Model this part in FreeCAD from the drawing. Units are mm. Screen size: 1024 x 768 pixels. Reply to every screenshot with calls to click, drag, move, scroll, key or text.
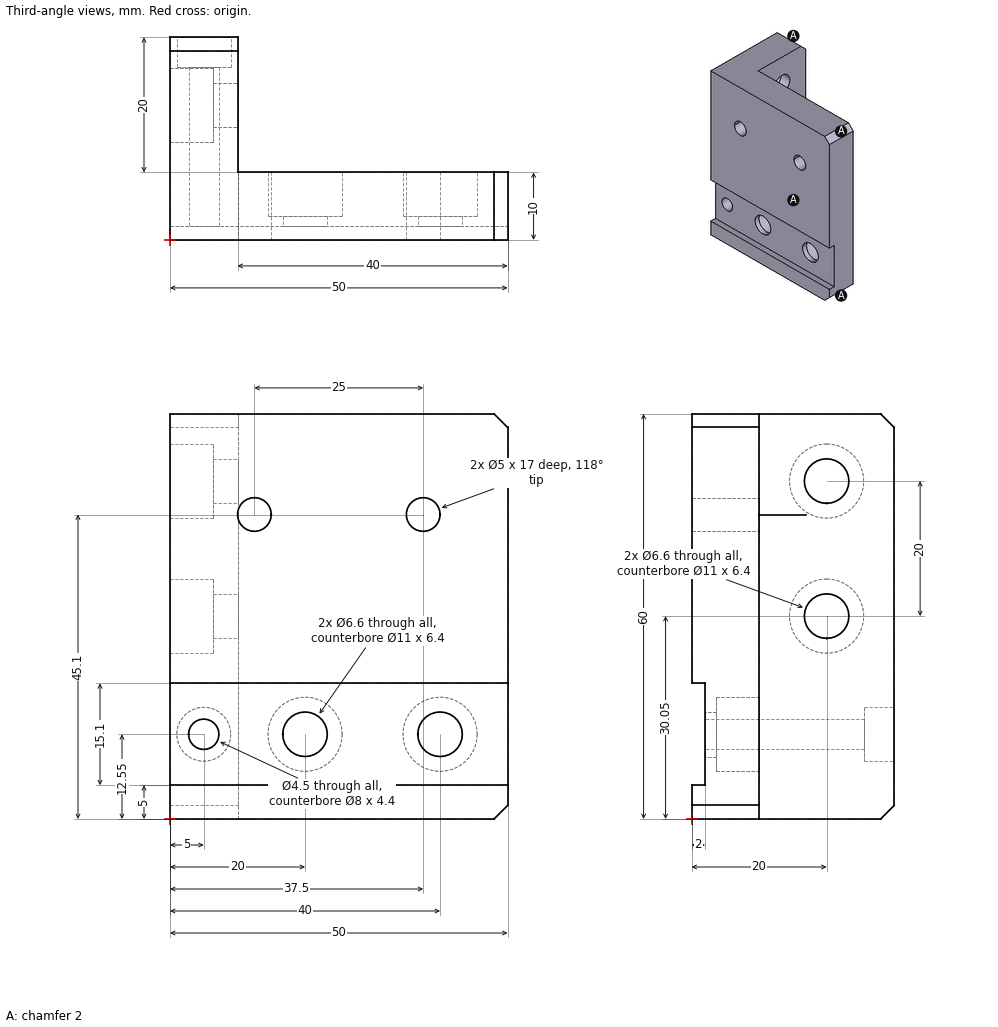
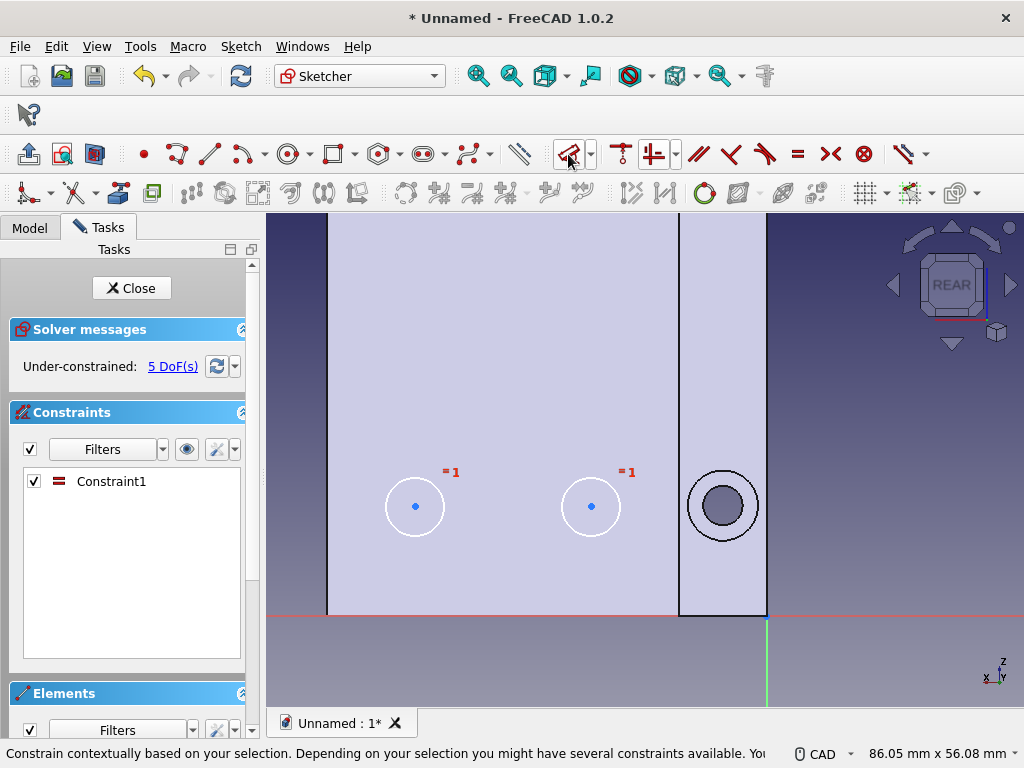
click(611, 486)
click(633, 463)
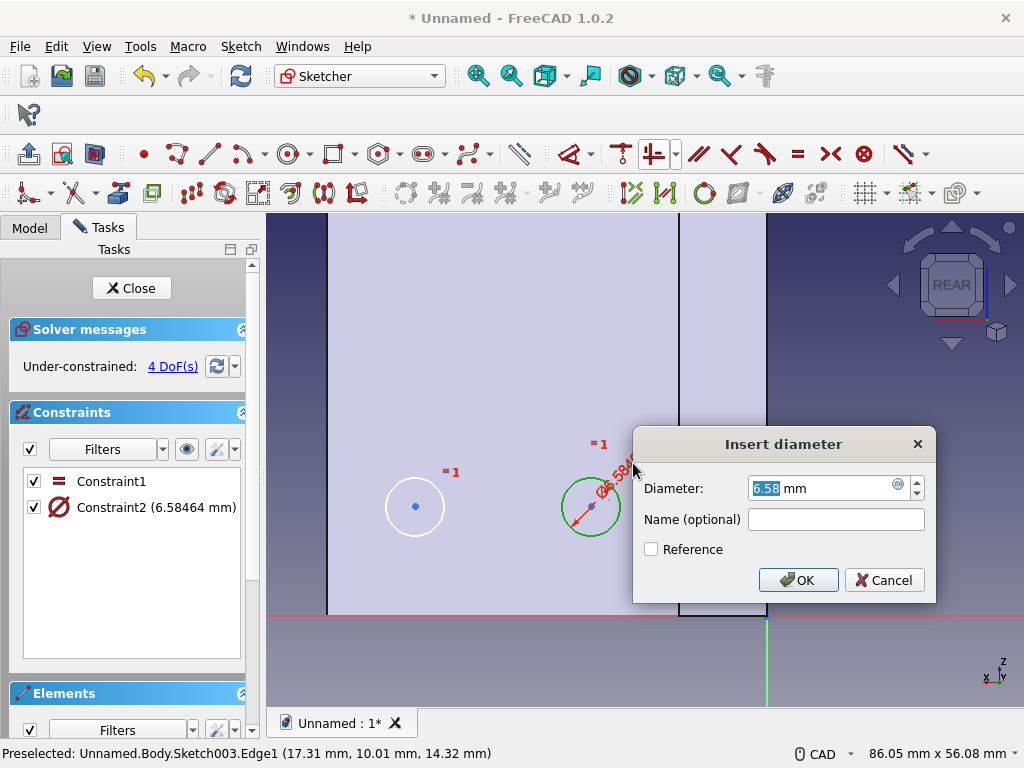
text(6.6)
key(Return)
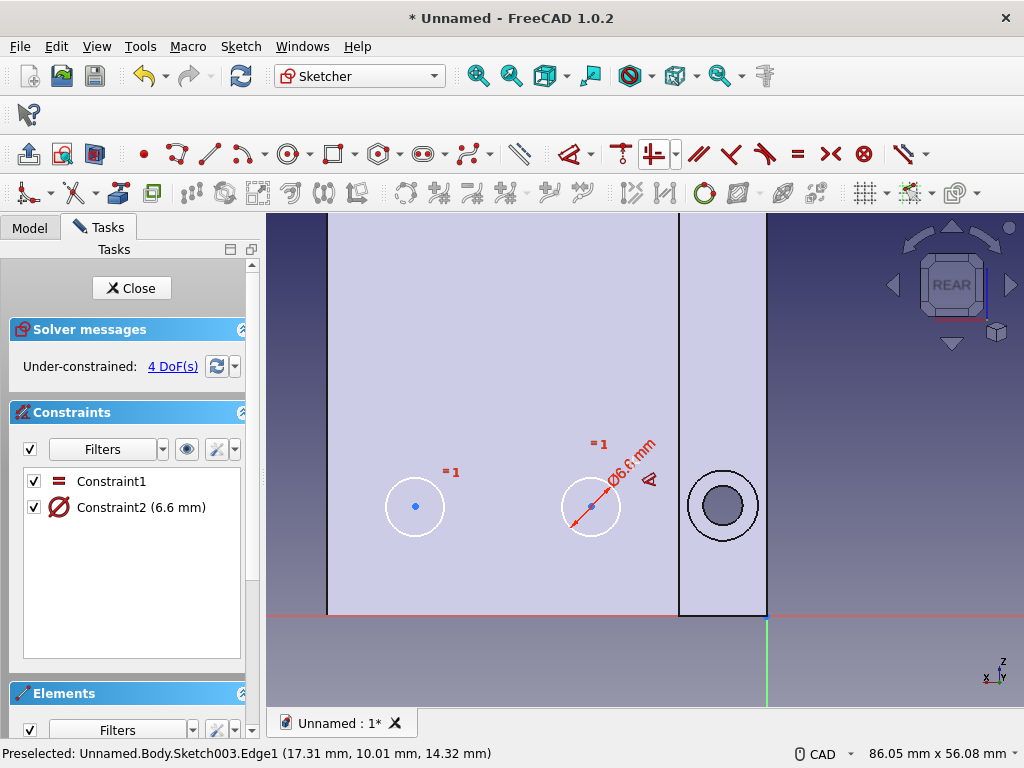
click(591, 507)
click(679, 650)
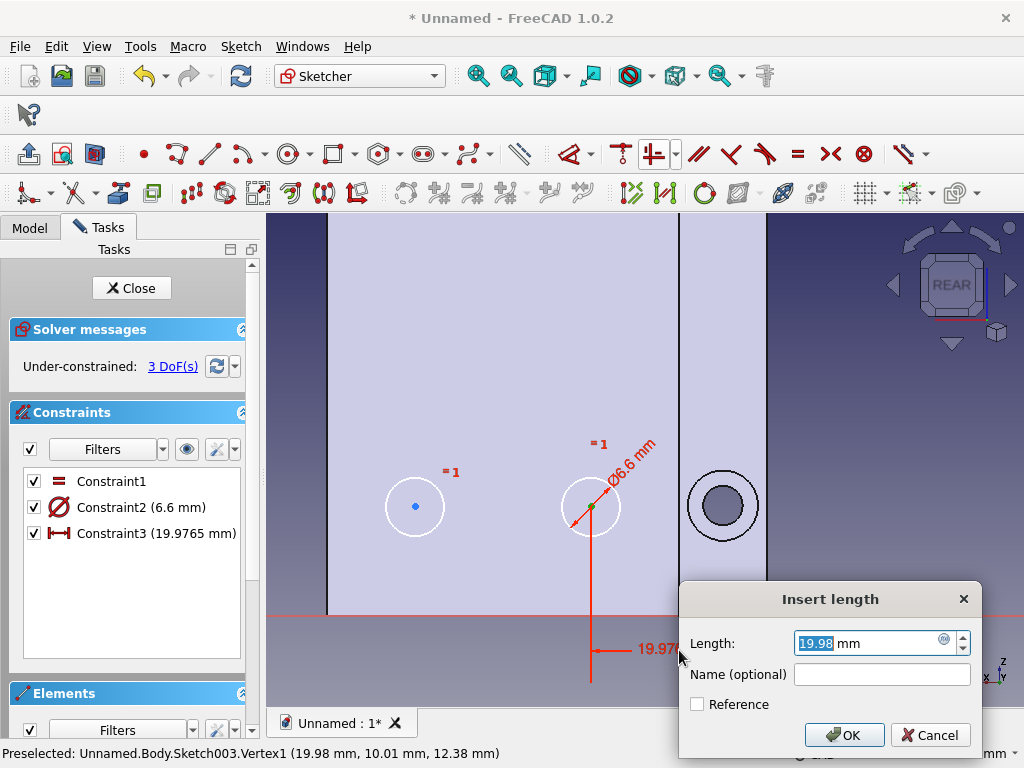
text(20)
key(Return)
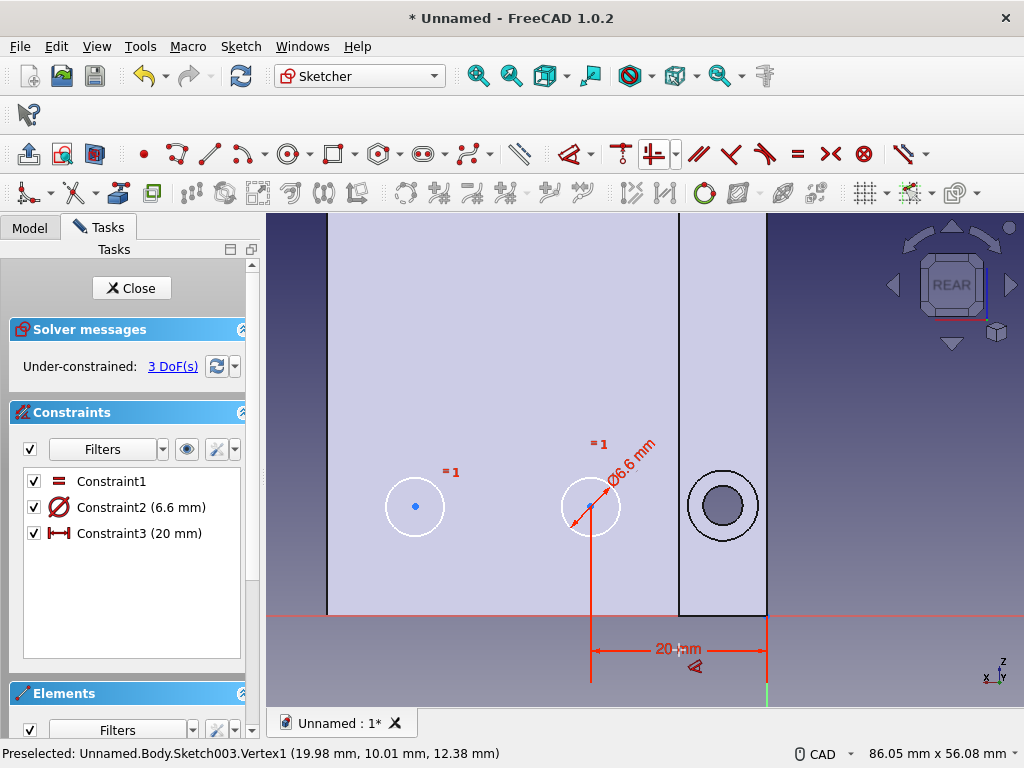
click(415, 507)
click(591, 650)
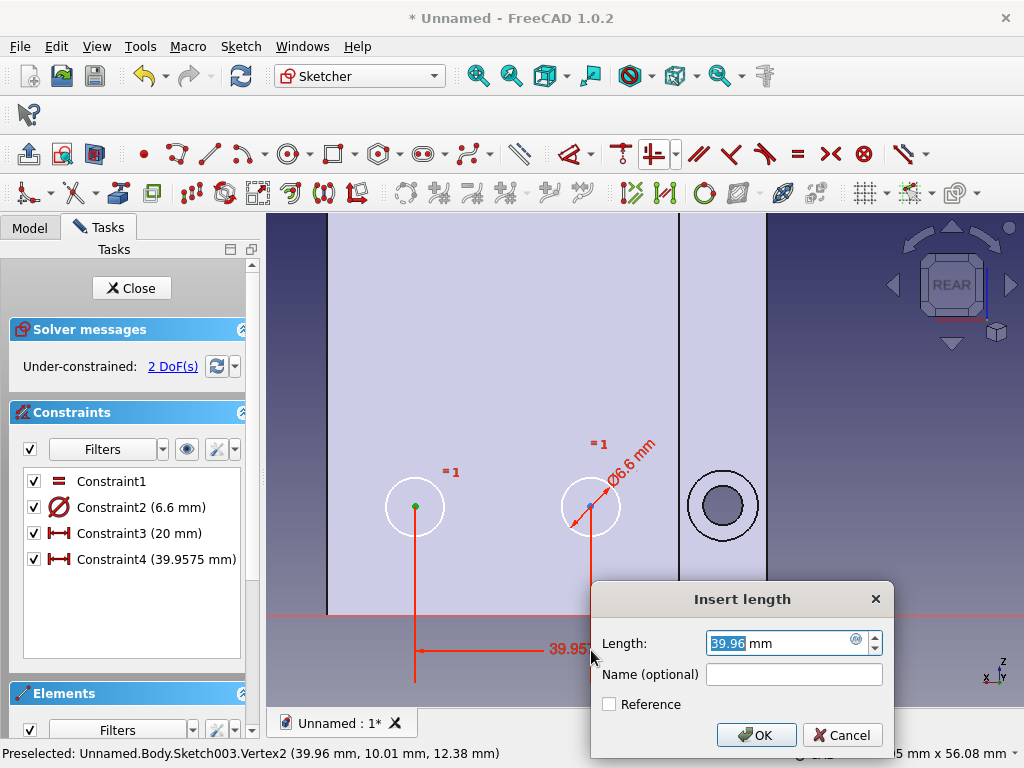
text(40)
key(Return)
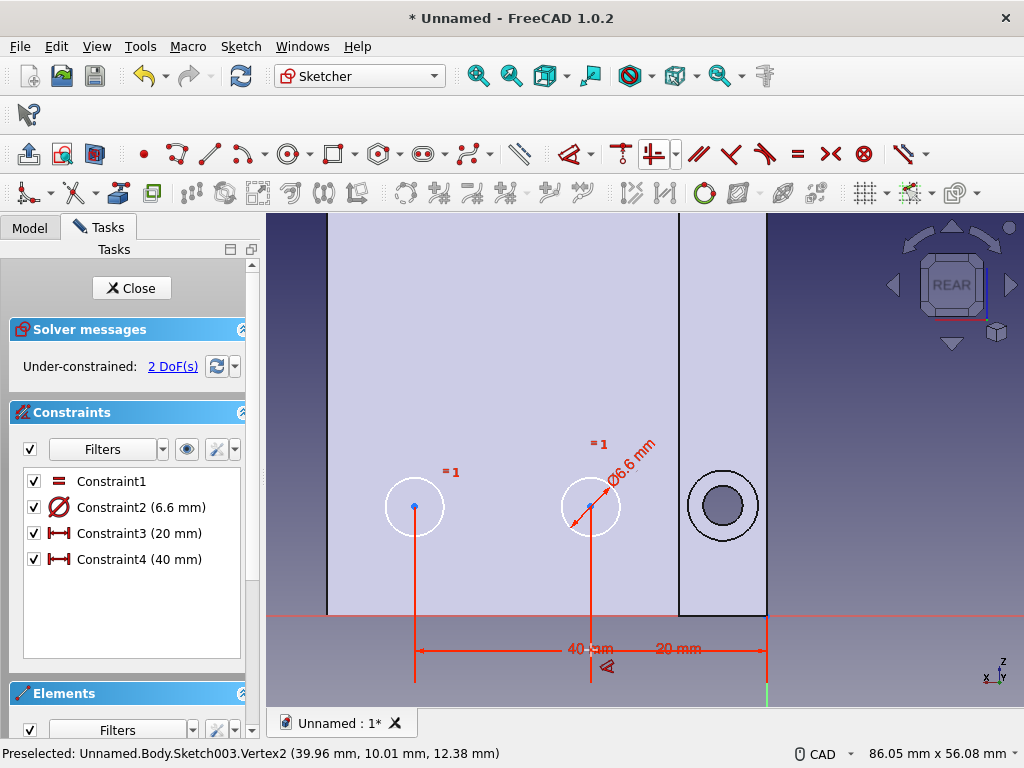
click(591, 507)
click(801, 562)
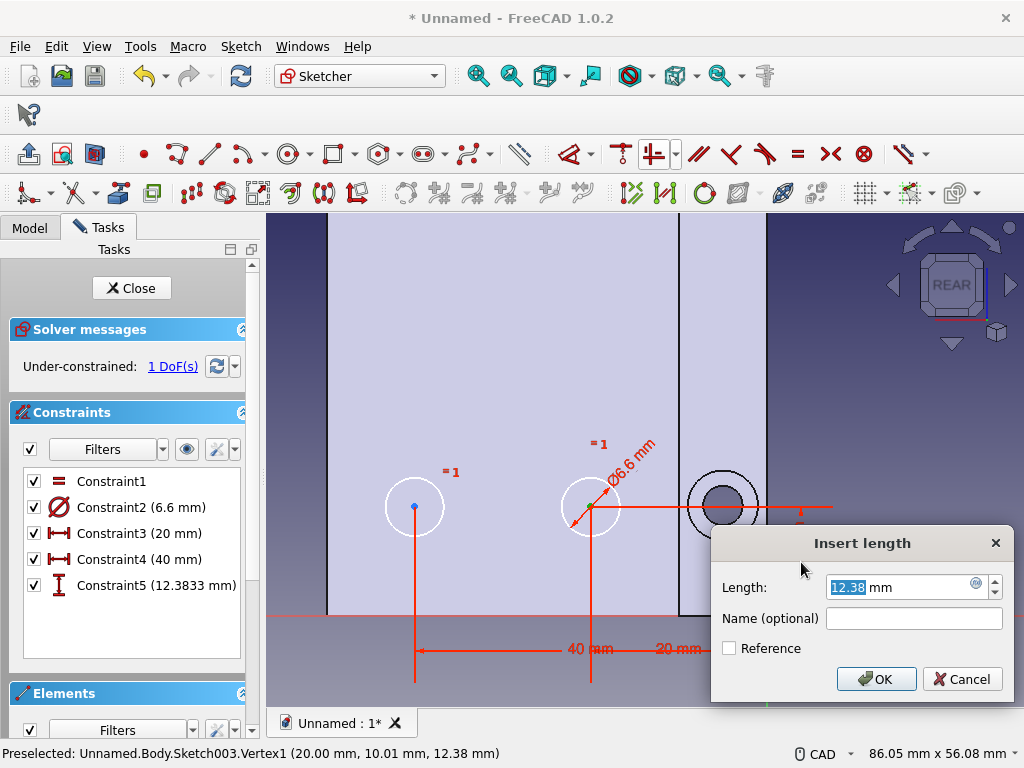
text(12.55)
key(Return)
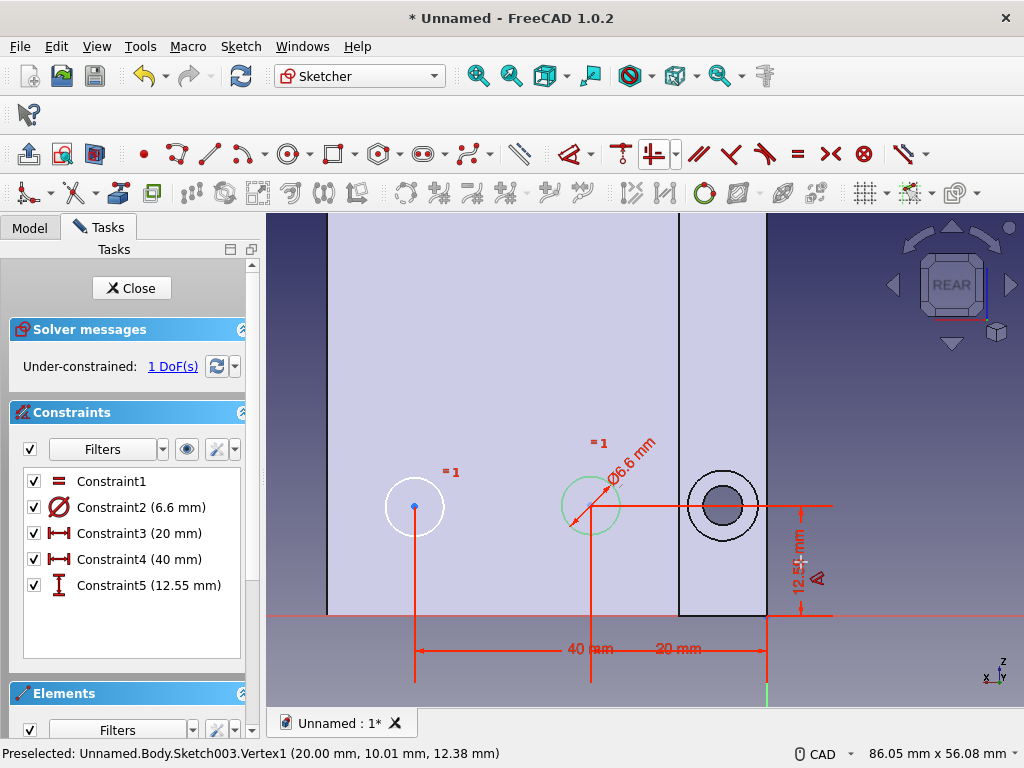
click(415, 507)
click(801, 536)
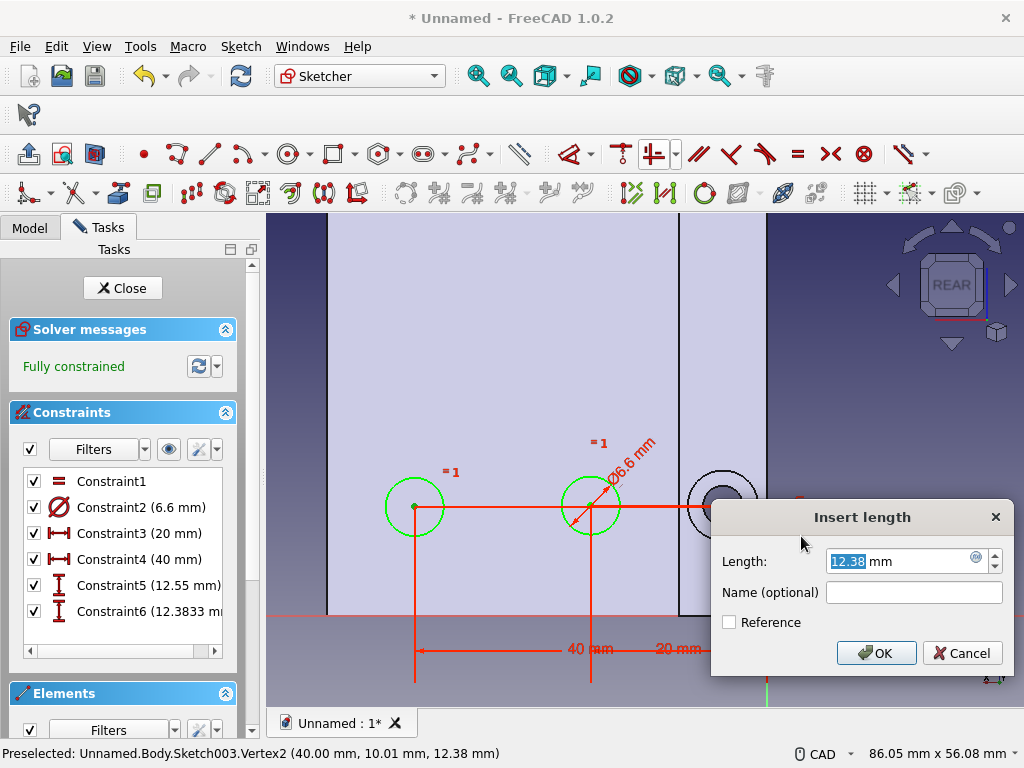
text(12.55)
key(Return)
key(Escape)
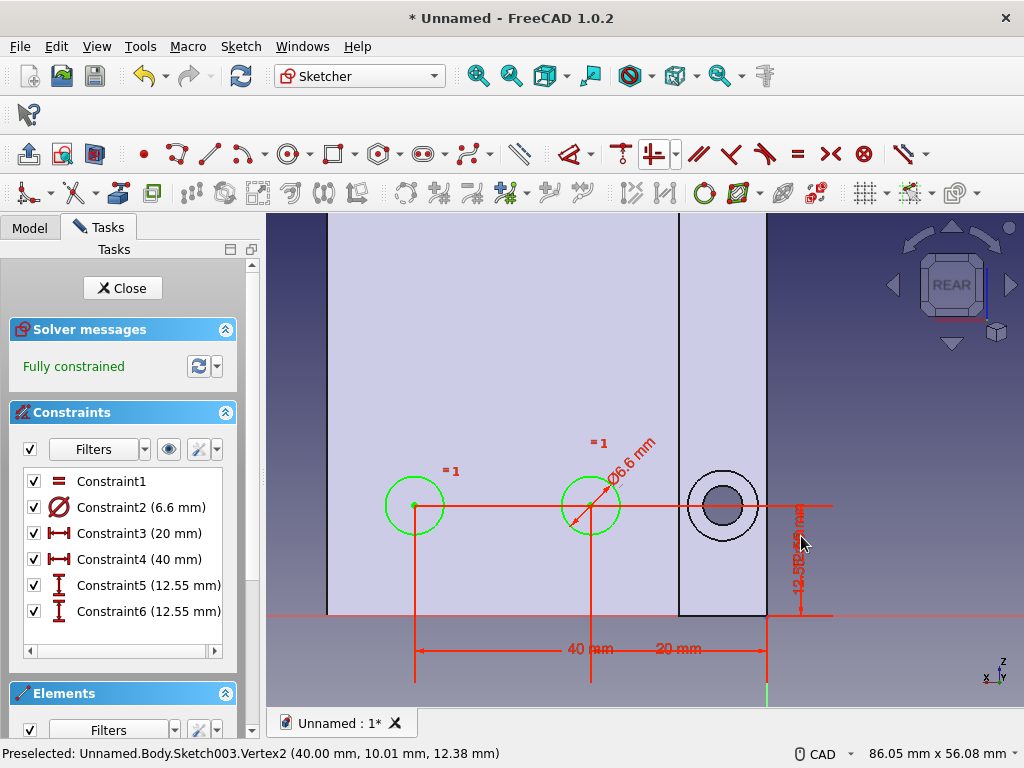
click(123, 288)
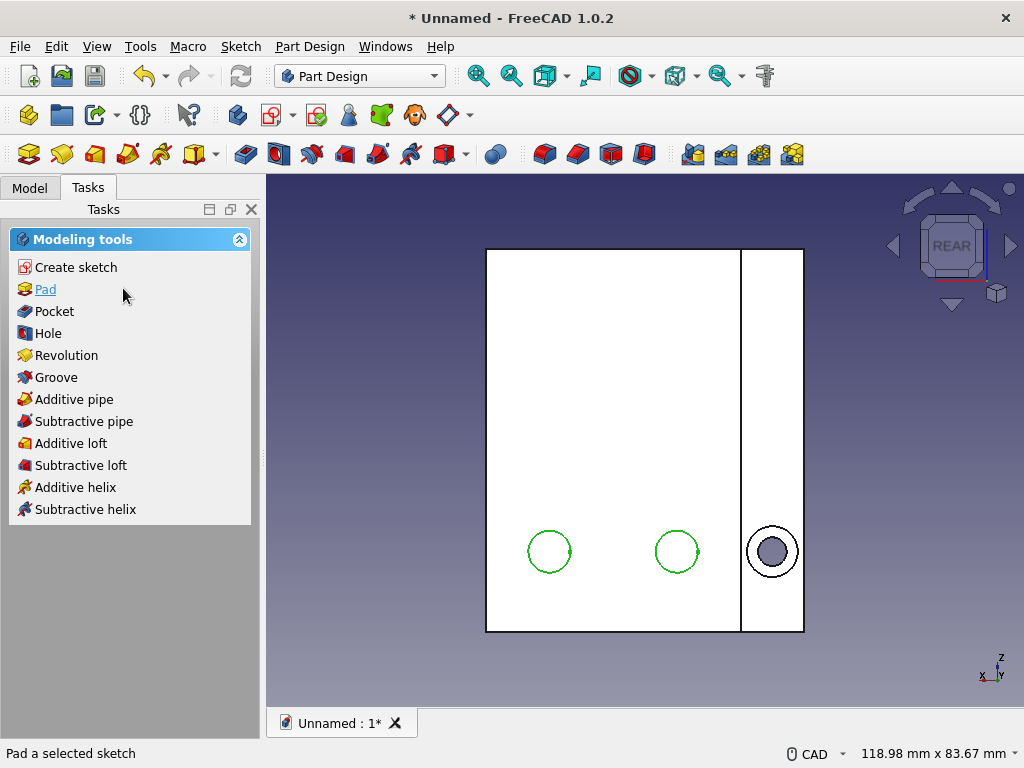
click(279, 154)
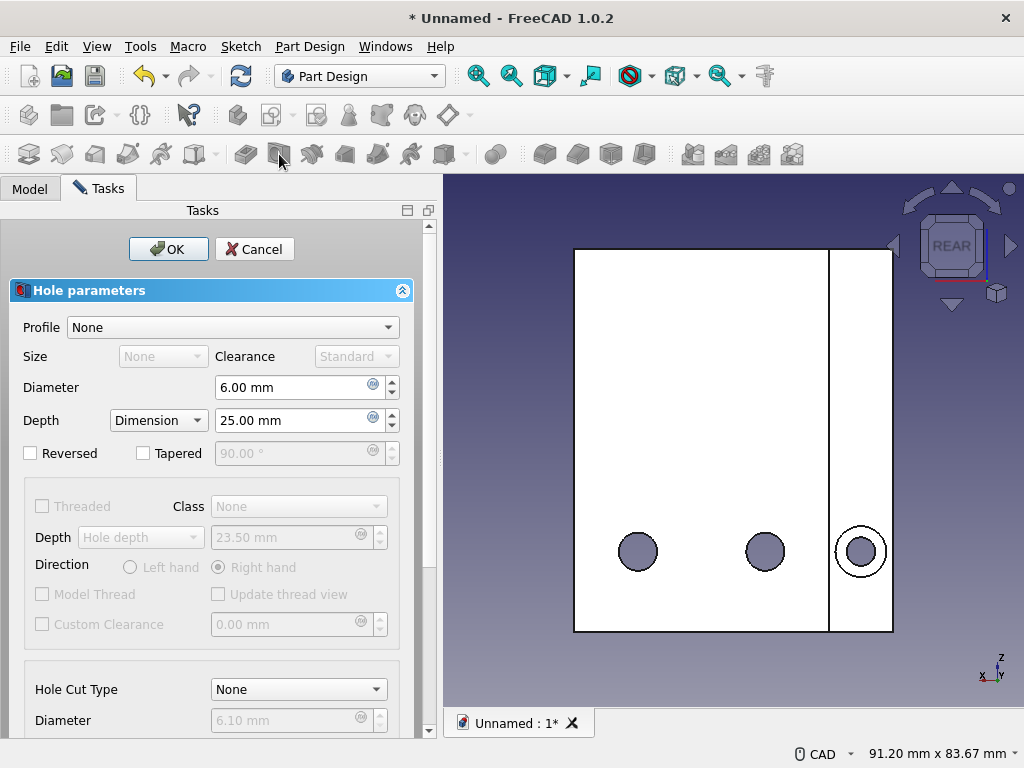
triple_click(300, 388)